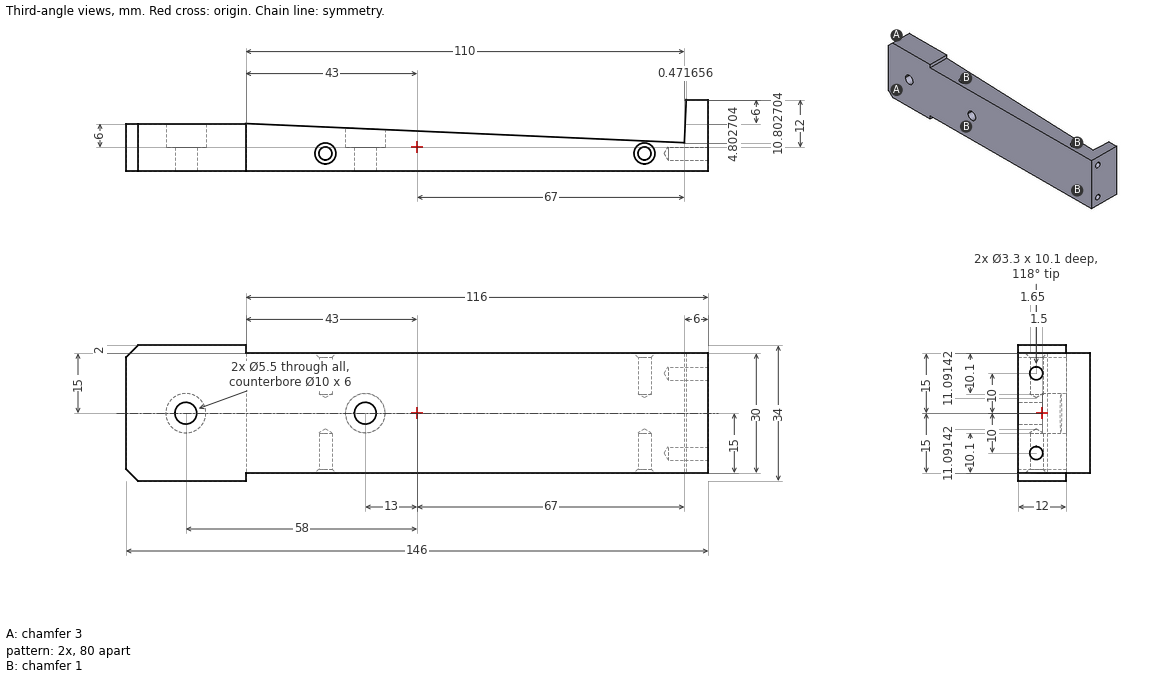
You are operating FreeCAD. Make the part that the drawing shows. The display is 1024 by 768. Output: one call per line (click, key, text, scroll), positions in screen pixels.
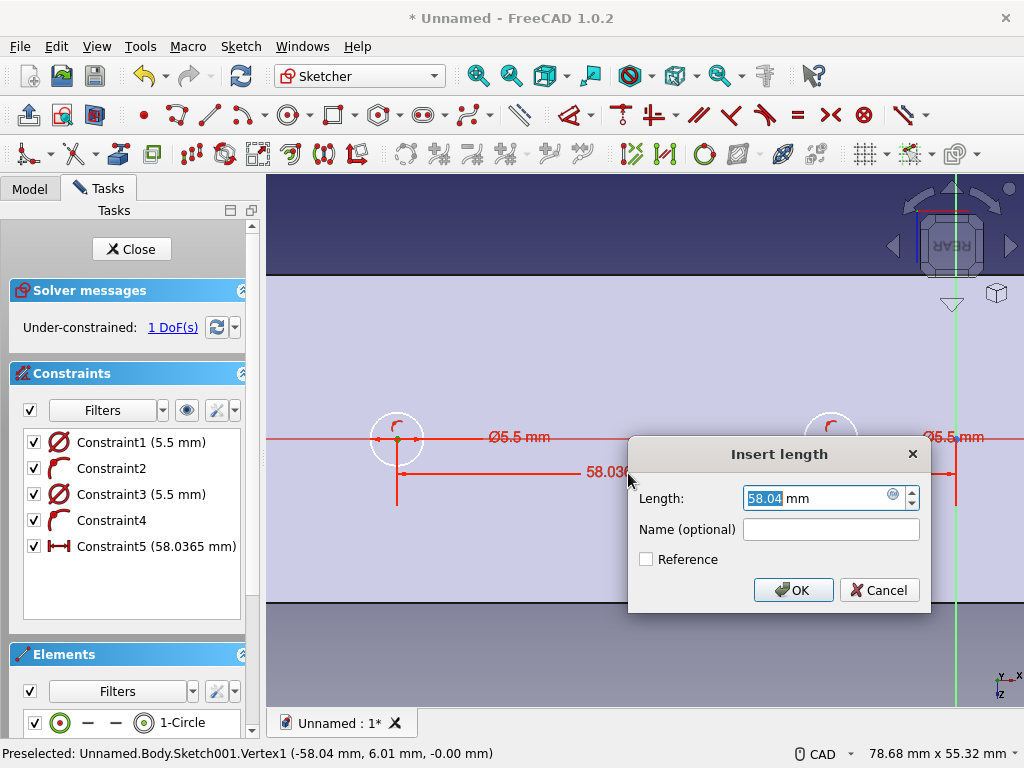
text(58)
key(Return)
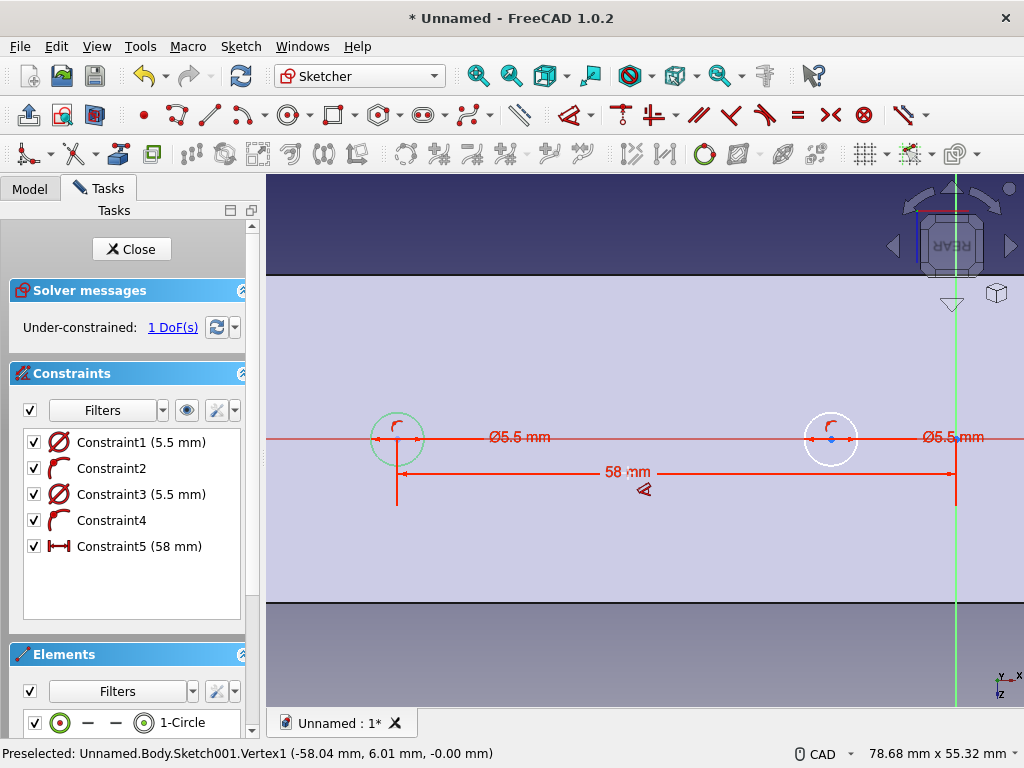
click(831, 439)
click(851, 473)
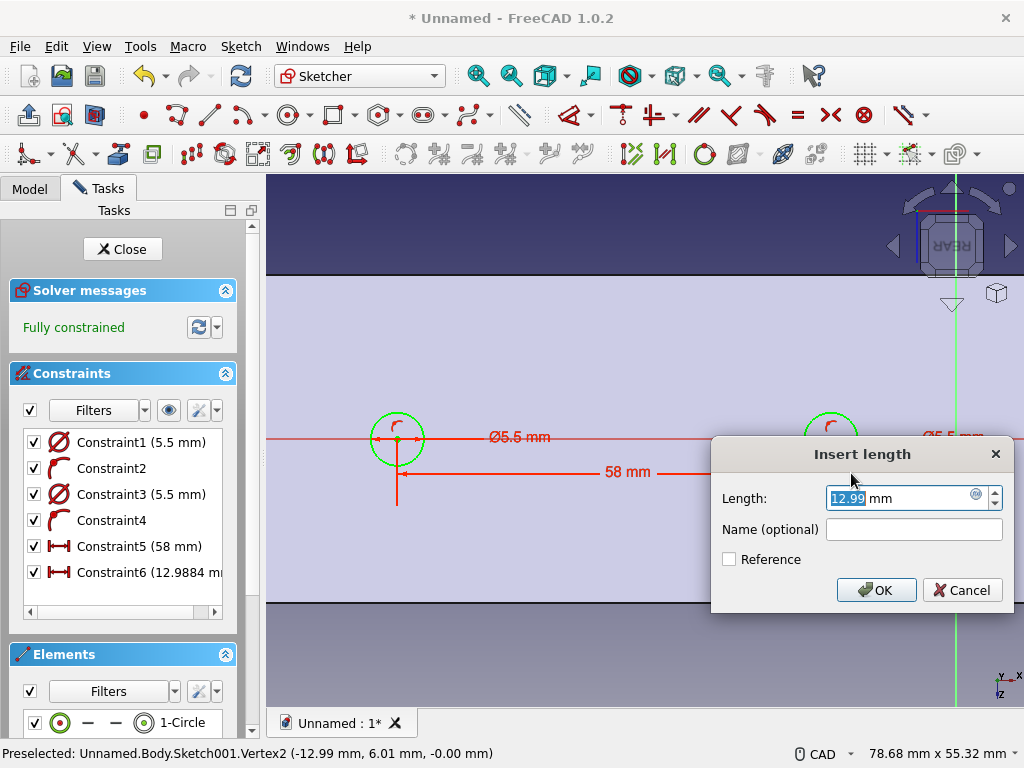
text(13)
key(Return)
key(Escape)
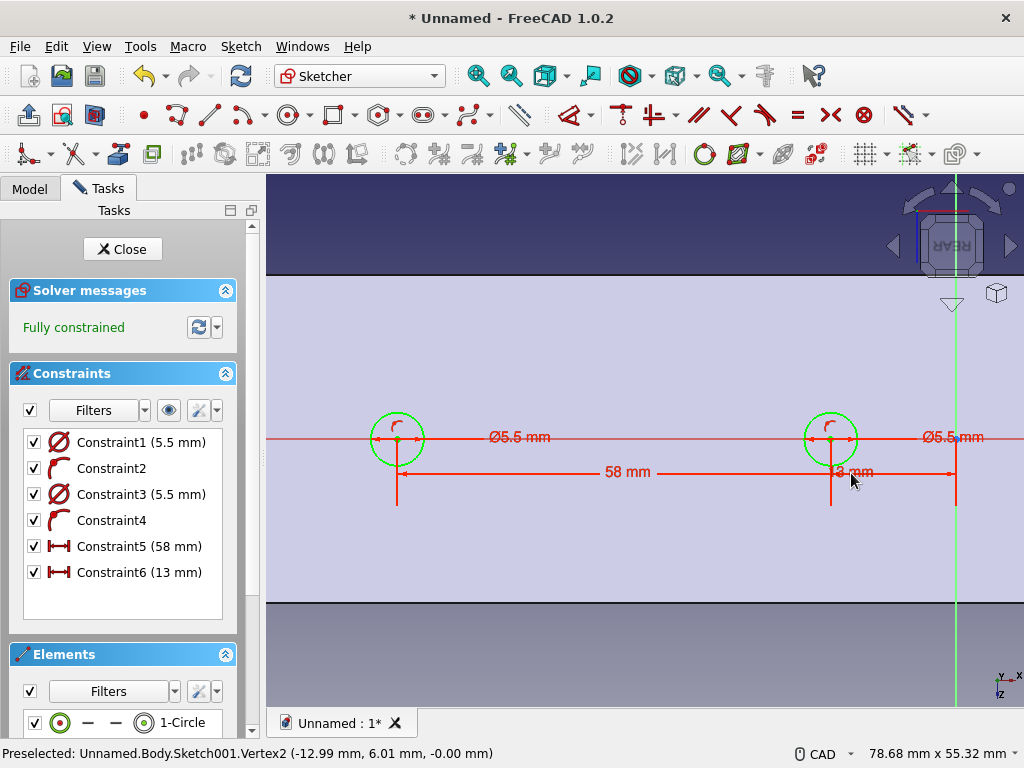
click(123, 249)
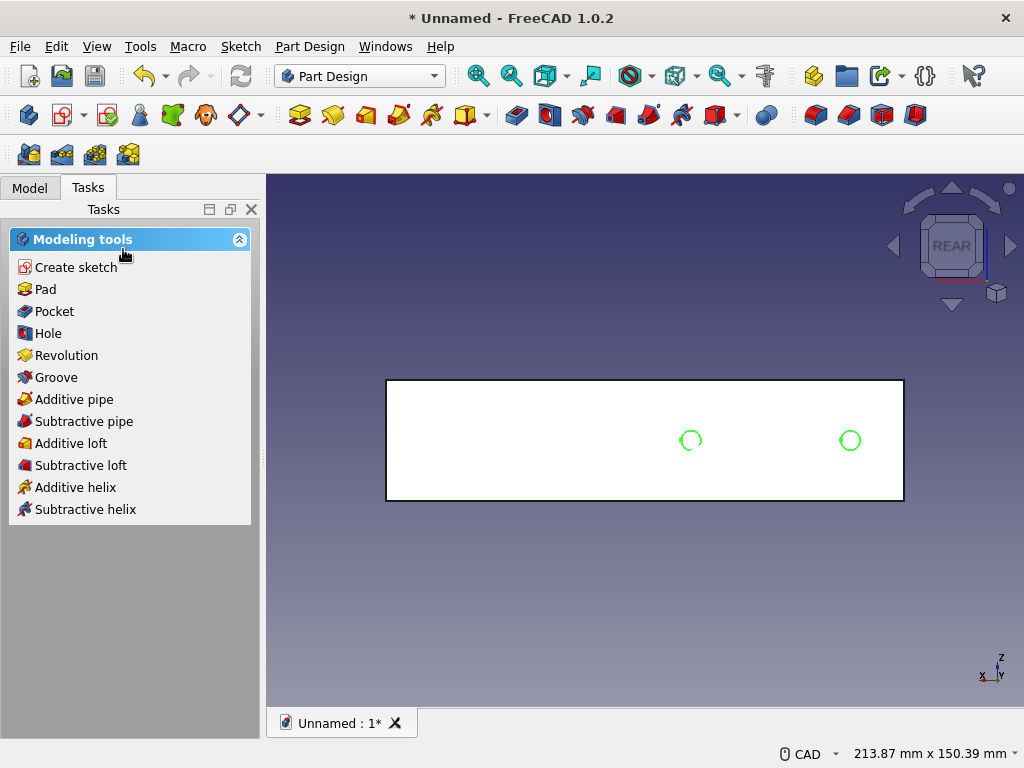
click(550, 116)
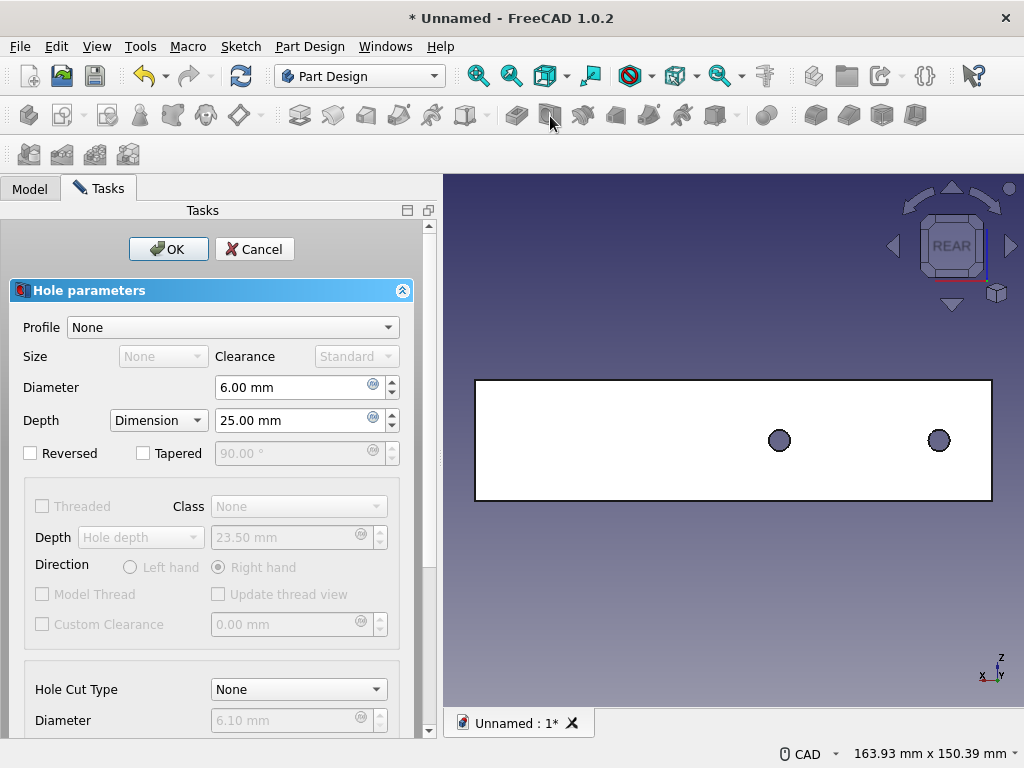
triple_click(300, 388)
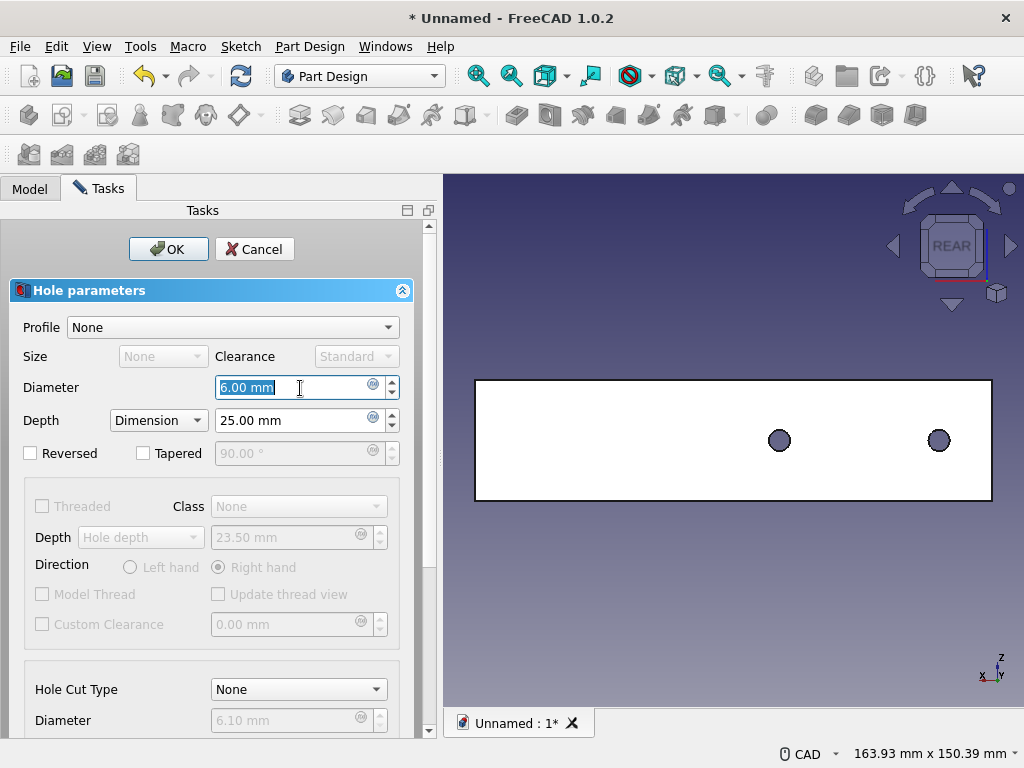
text(5.5)
key(Tab)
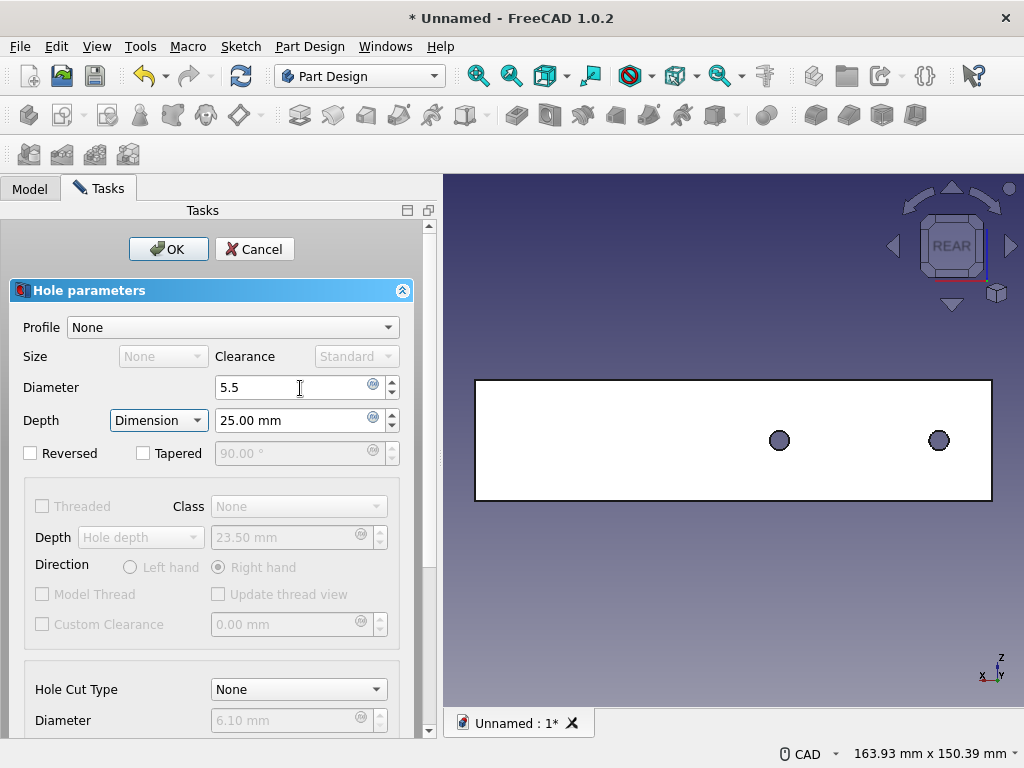
click(160, 420)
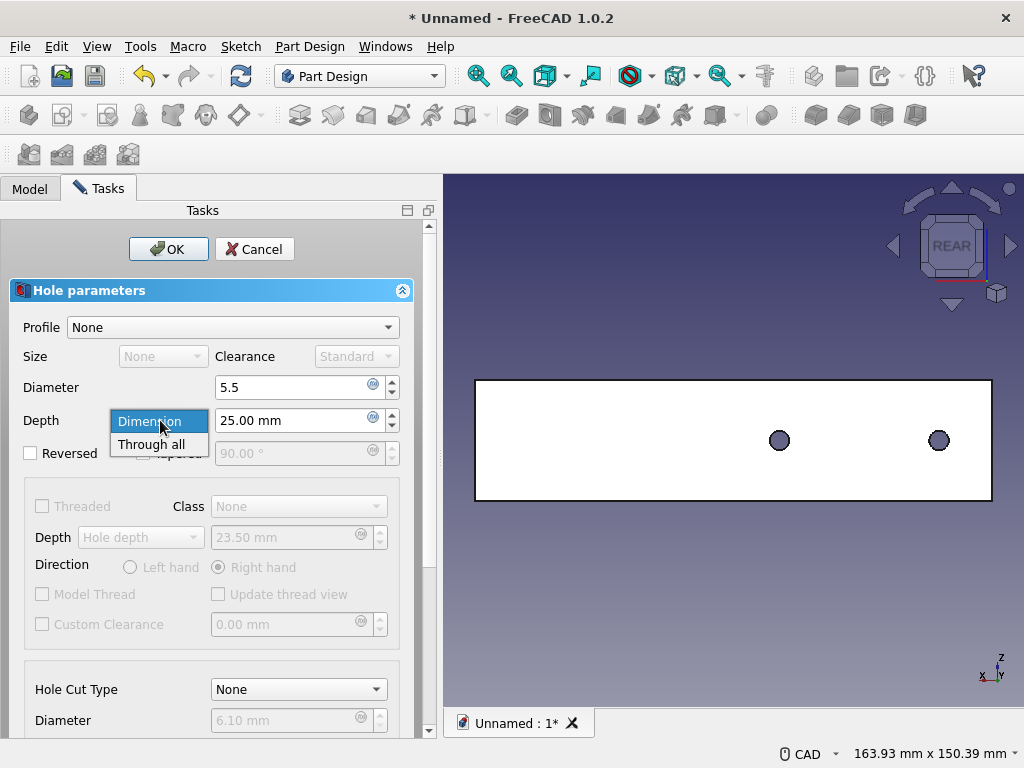
click(158, 444)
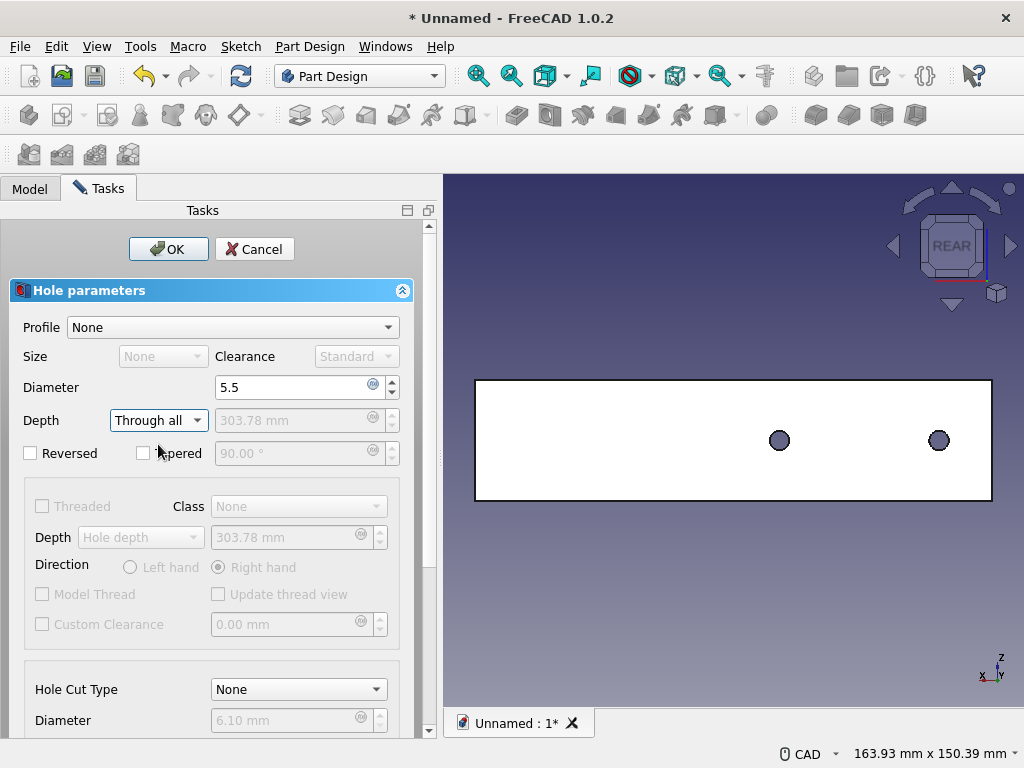
click(300, 690)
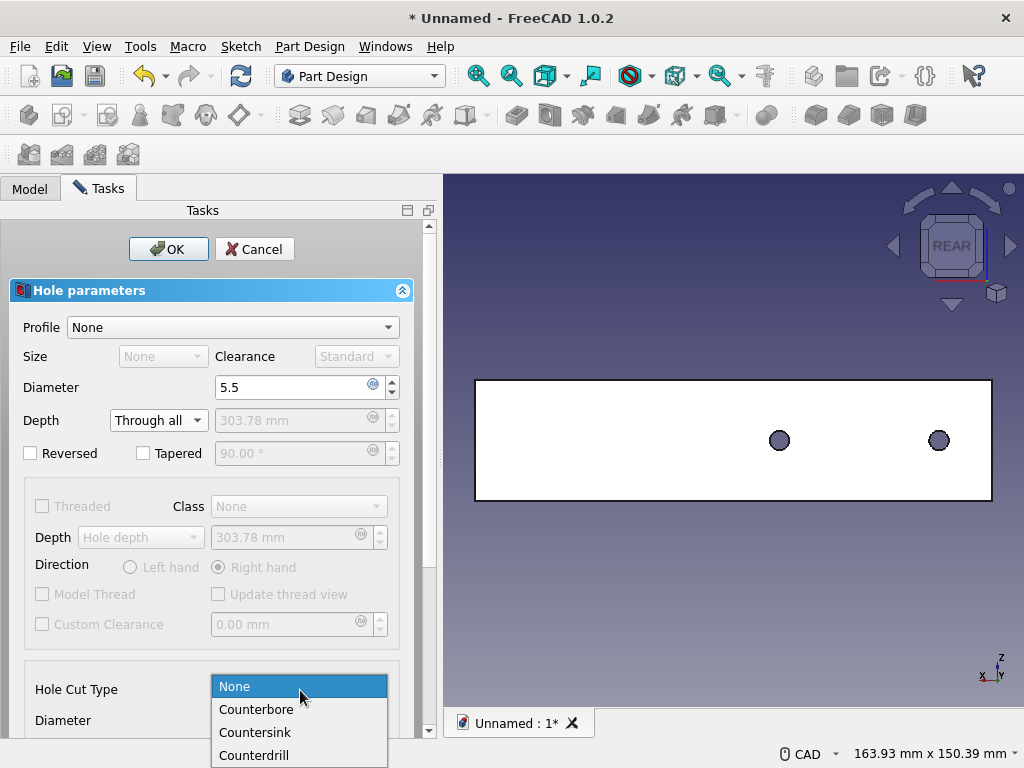
click(298, 710)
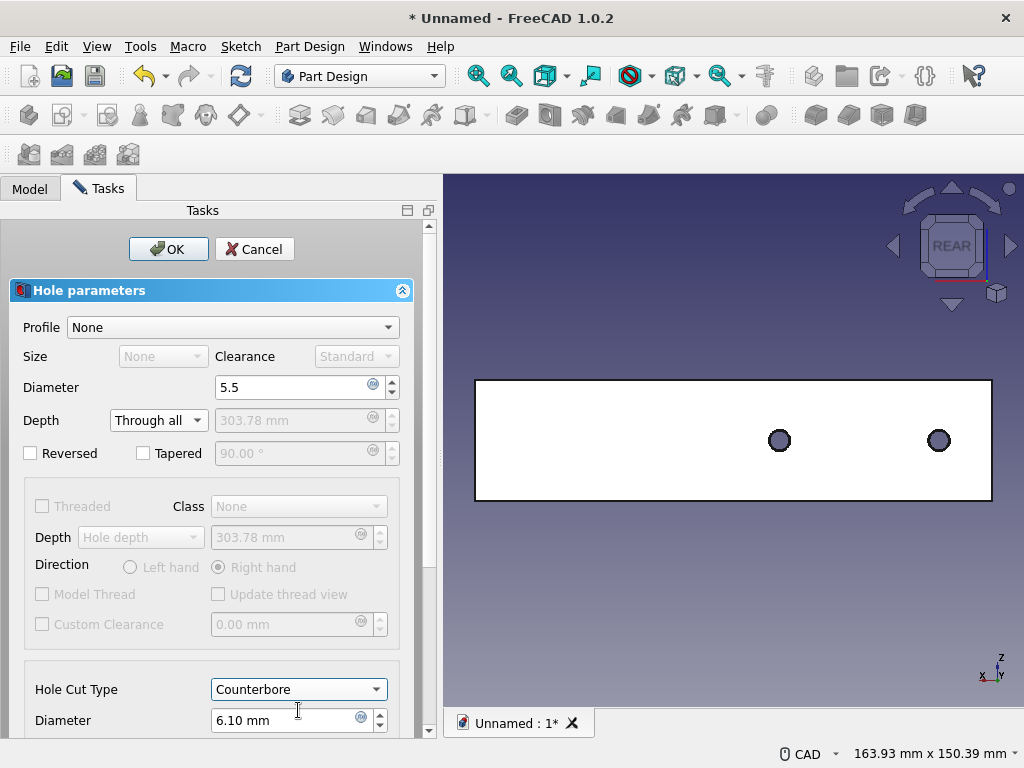
triple_click(292, 720)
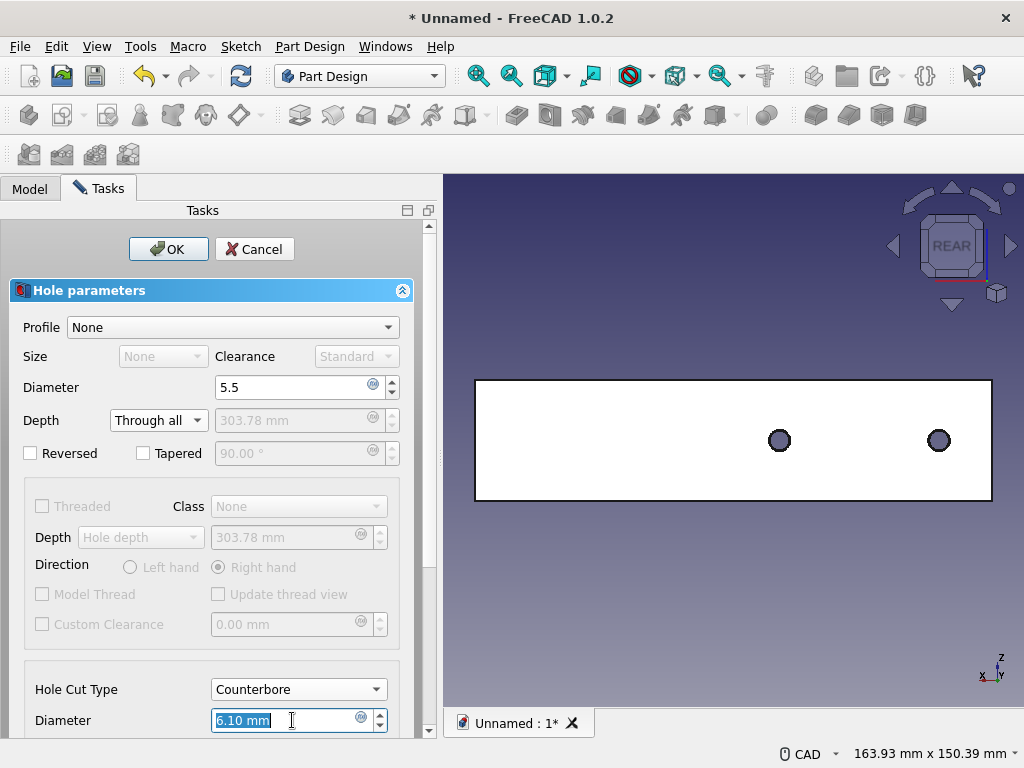
text(10)
key(Tab)